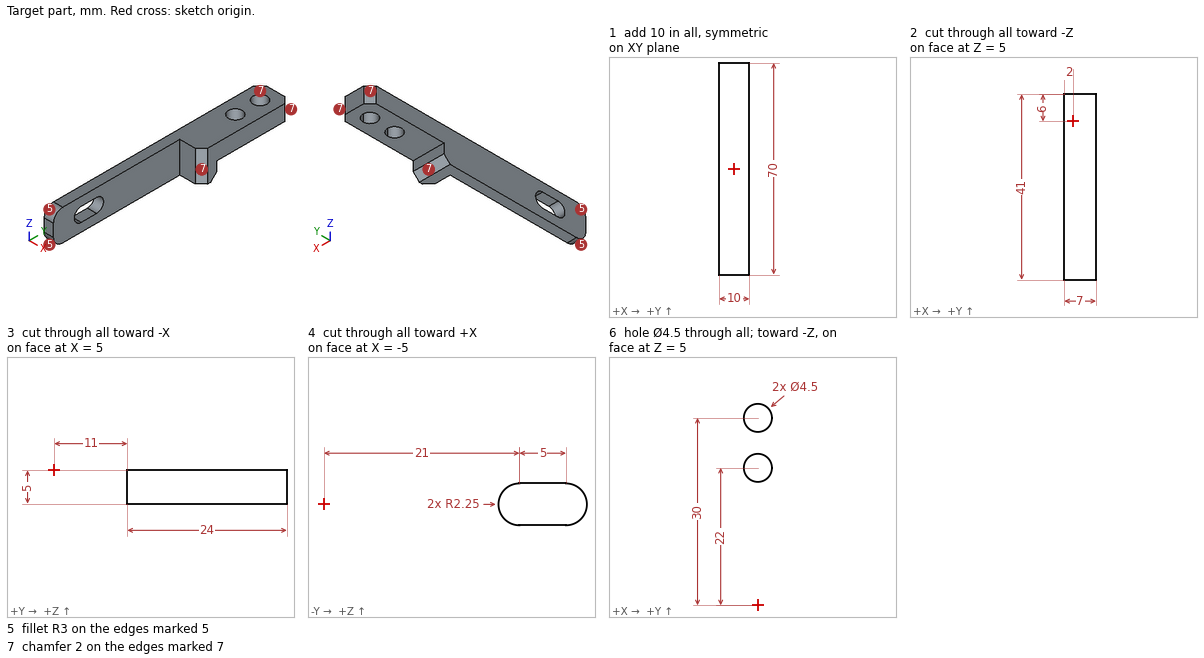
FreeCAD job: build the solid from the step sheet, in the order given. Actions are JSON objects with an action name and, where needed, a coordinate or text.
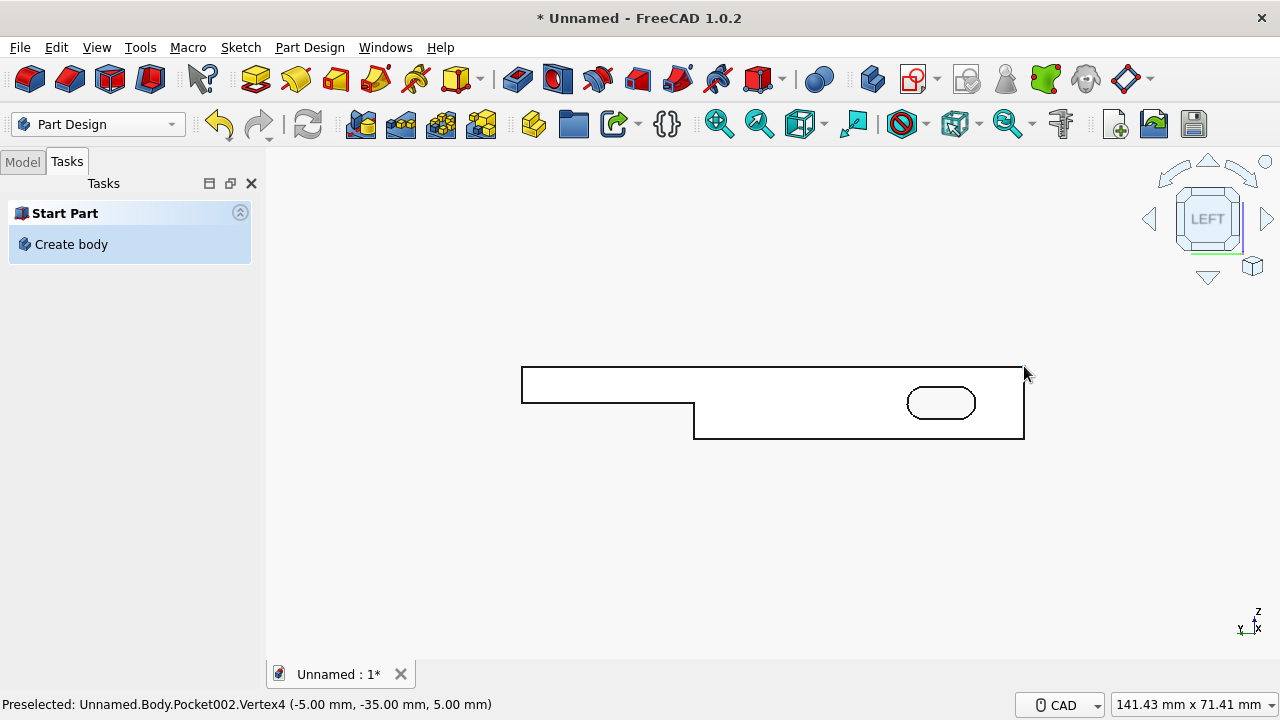
{"action": "key", "text": "0"}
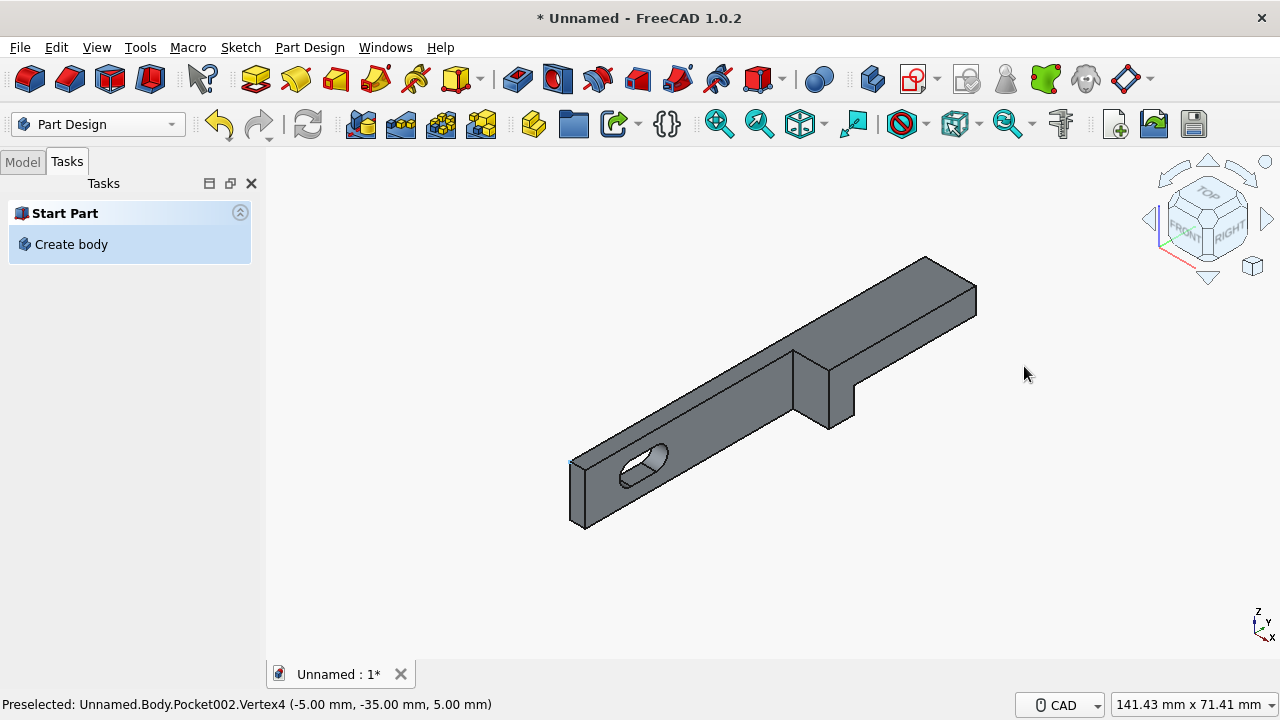
{"action": "left_click", "coordinate": [578, 465]}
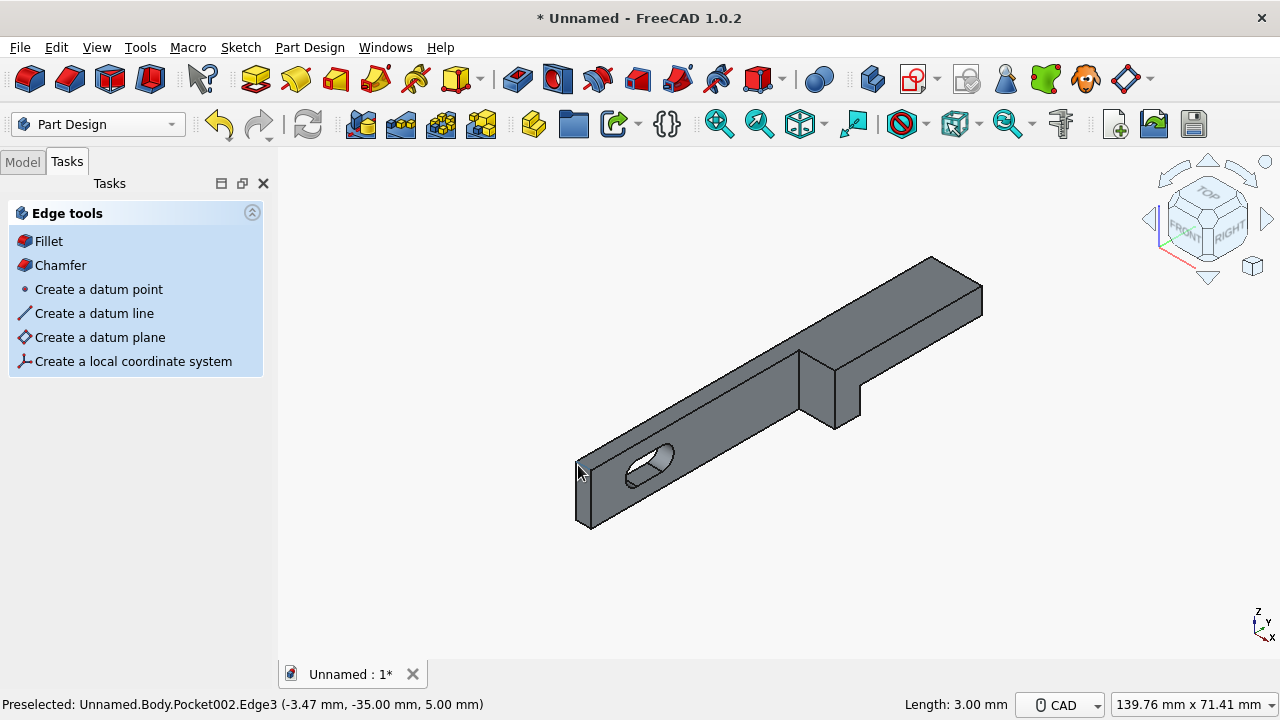
{"action": "scroll", "coordinate": [584, 523], "scroll_direction": "up", "scroll_amount": 4}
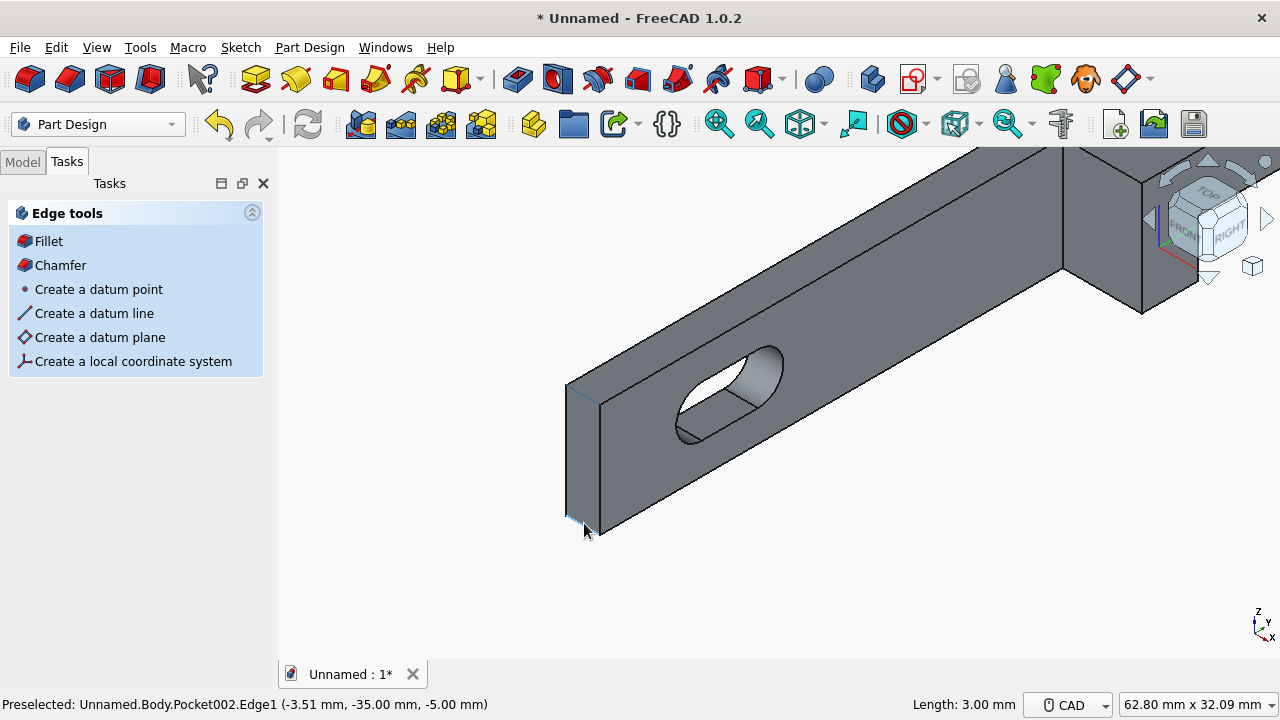
{"action": "key", "text": "v f"}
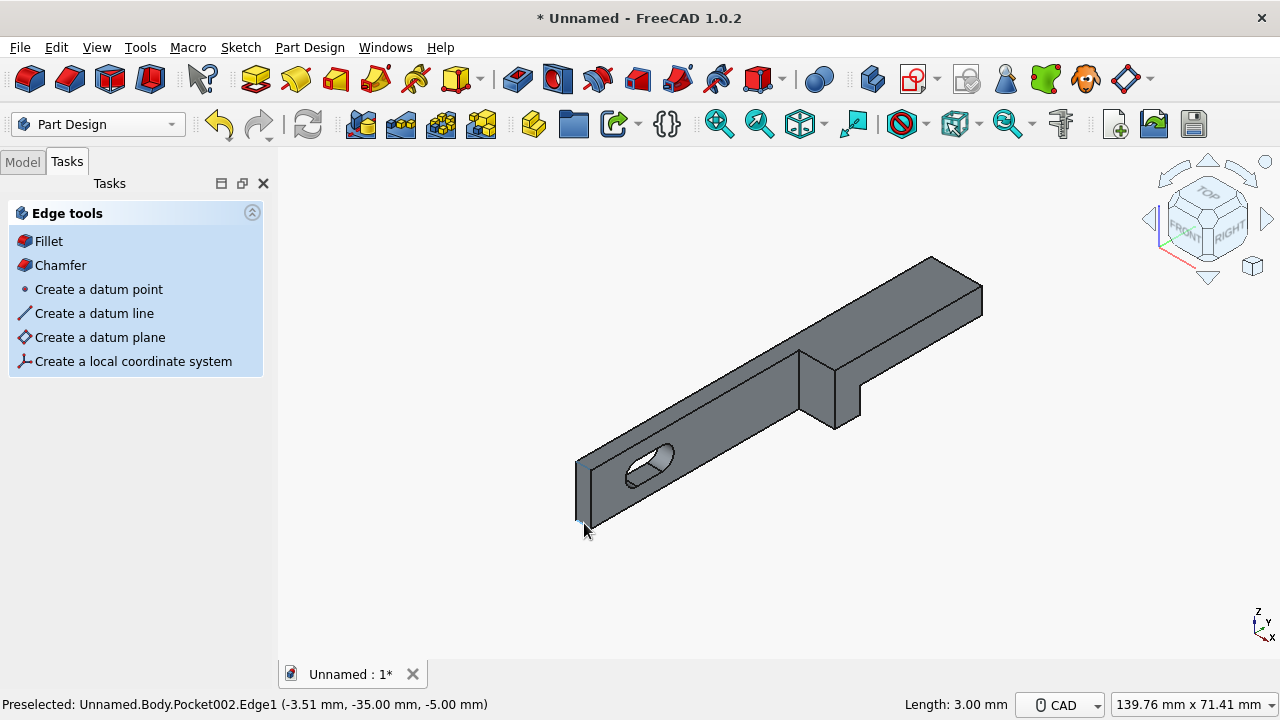
{"action": "key", "text": "2"}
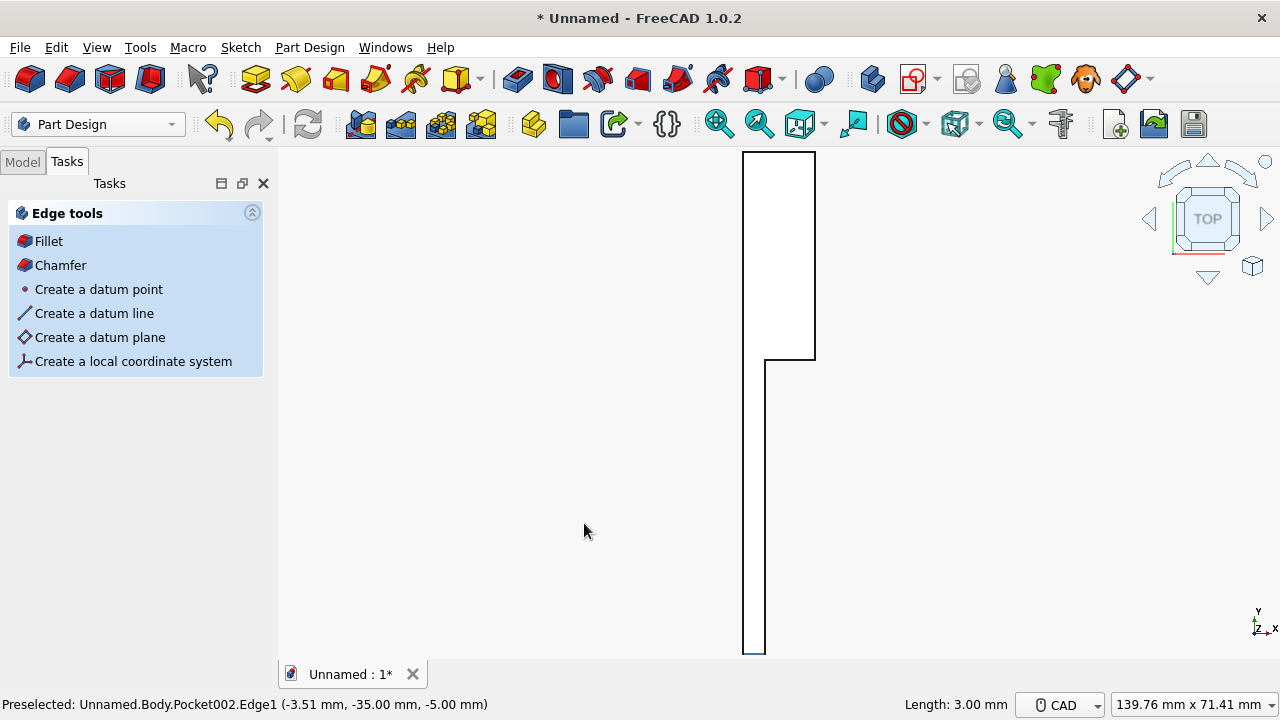
{"action": "key", "text": "1"}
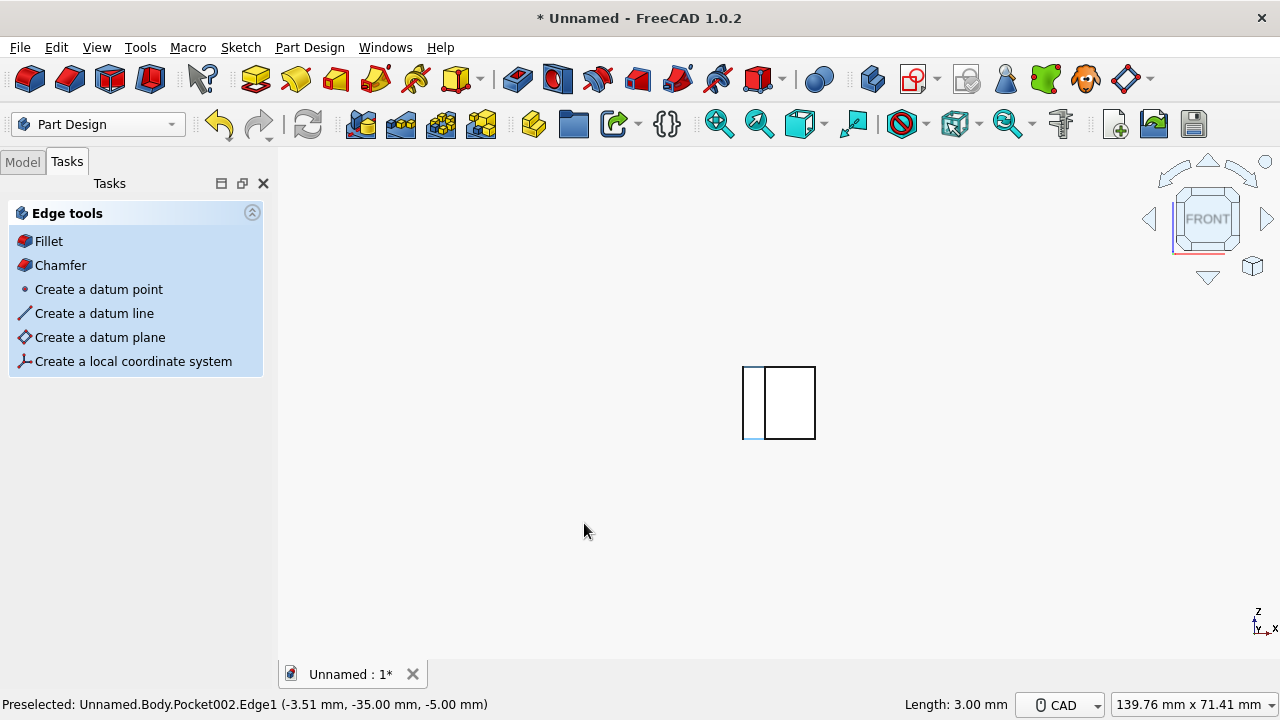
{"action": "key", "text": "v f"}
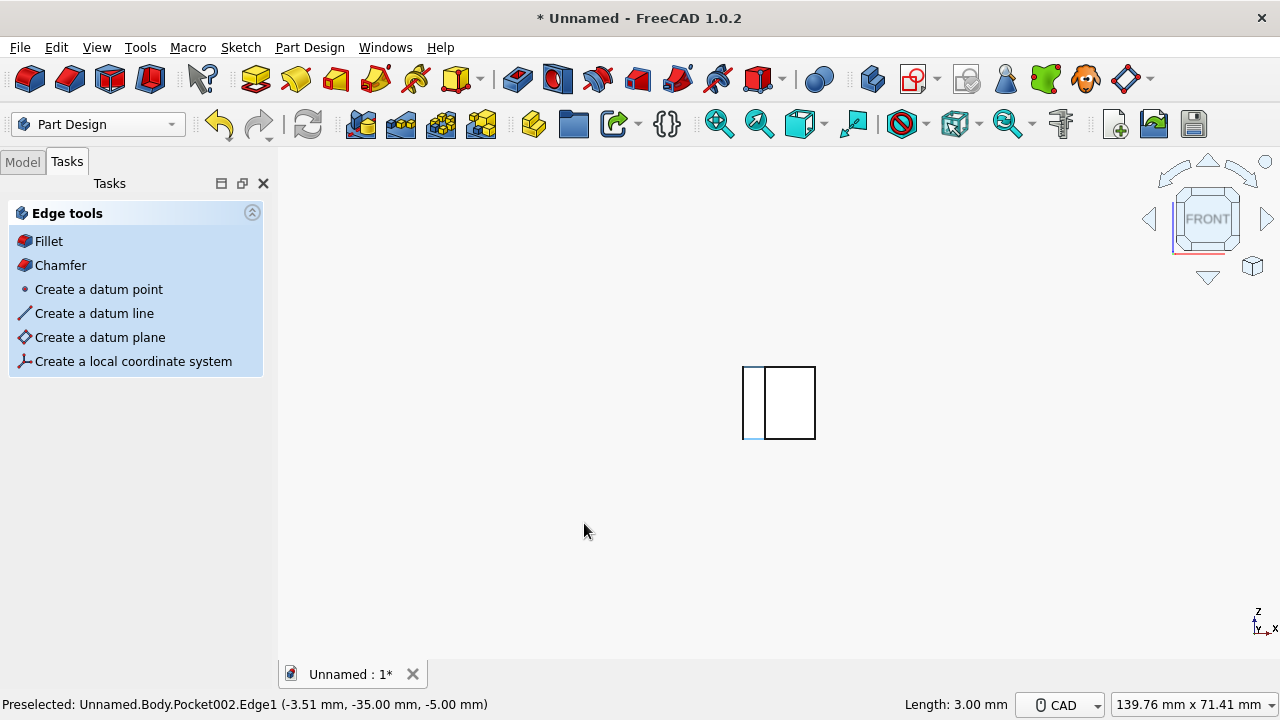
{"action": "left_click", "coordinate": [754, 438], "text": "ctrl"}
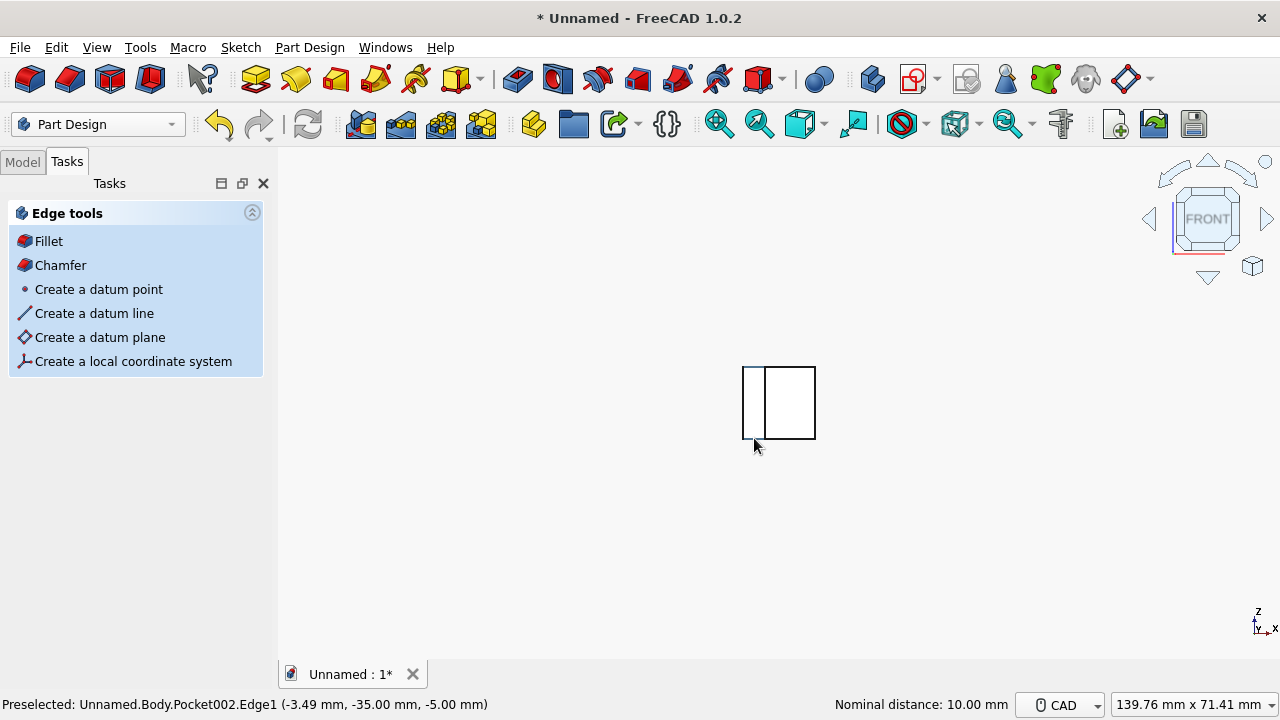
{"action": "left_click", "coordinate": [30, 80]}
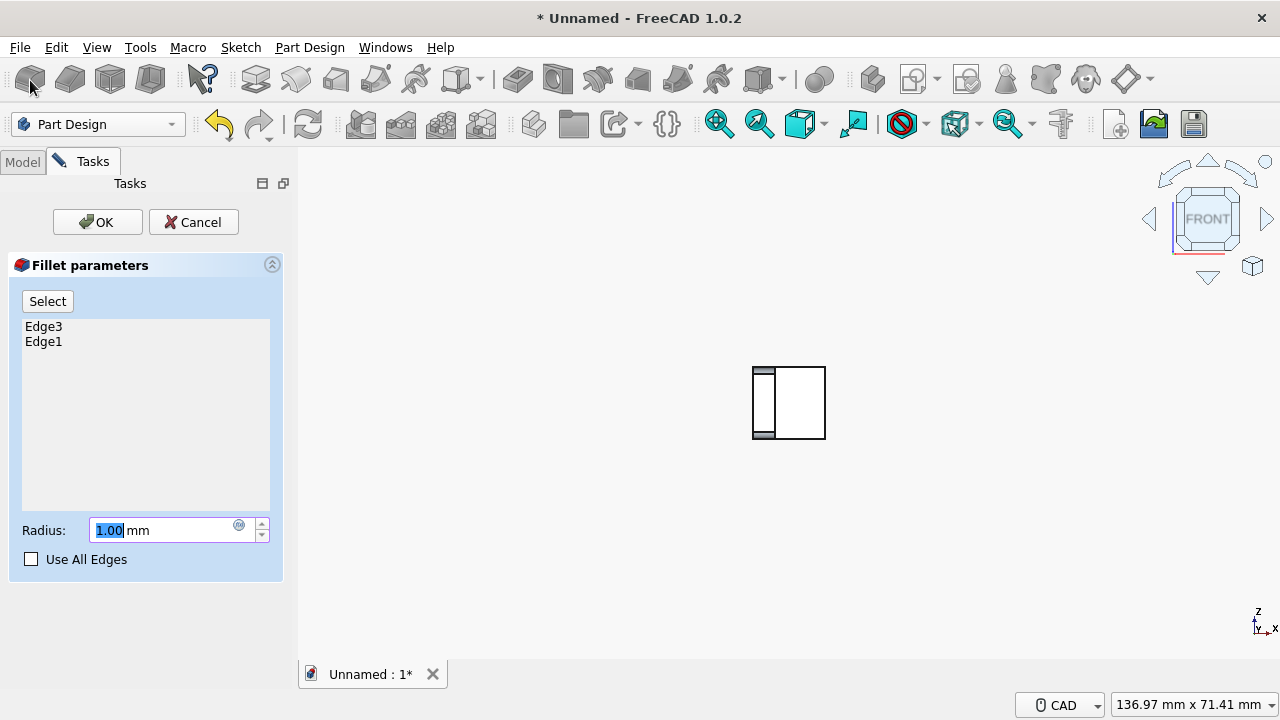
{"action": "type", "text": "3"}
{"action": "key", "text": "Tab"}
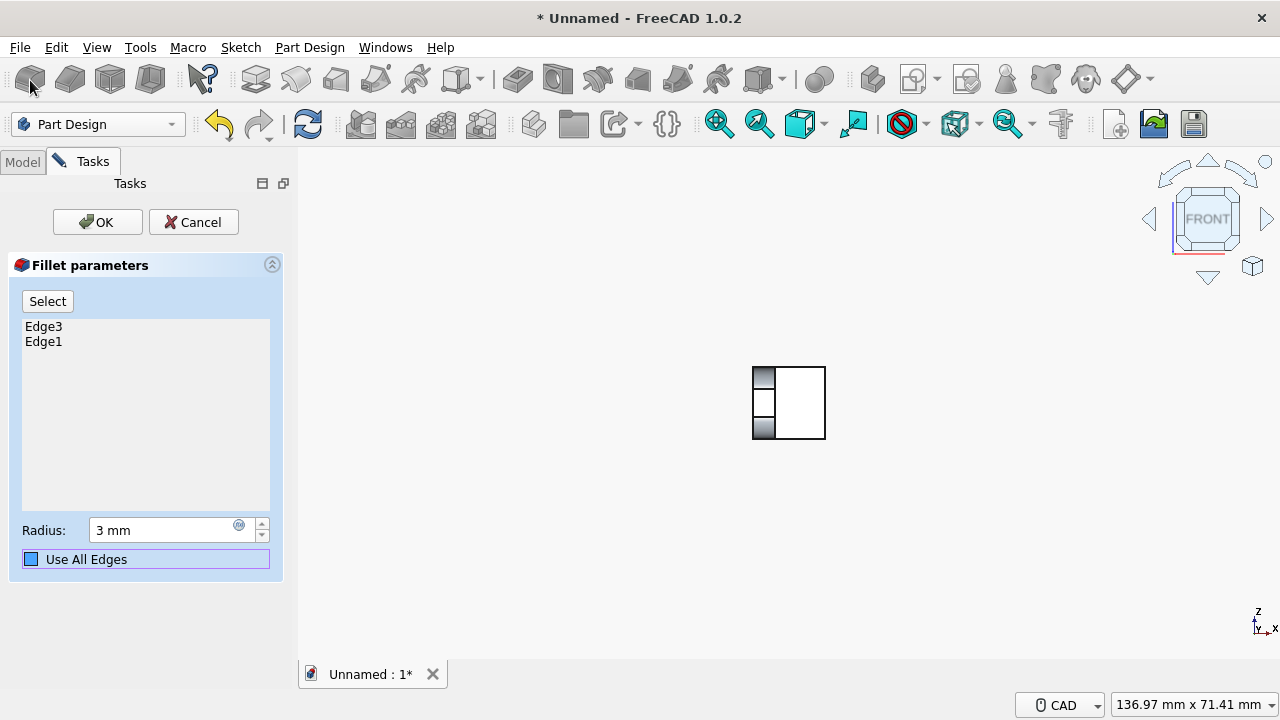
{"action": "left_click", "coordinate": [98, 222]}